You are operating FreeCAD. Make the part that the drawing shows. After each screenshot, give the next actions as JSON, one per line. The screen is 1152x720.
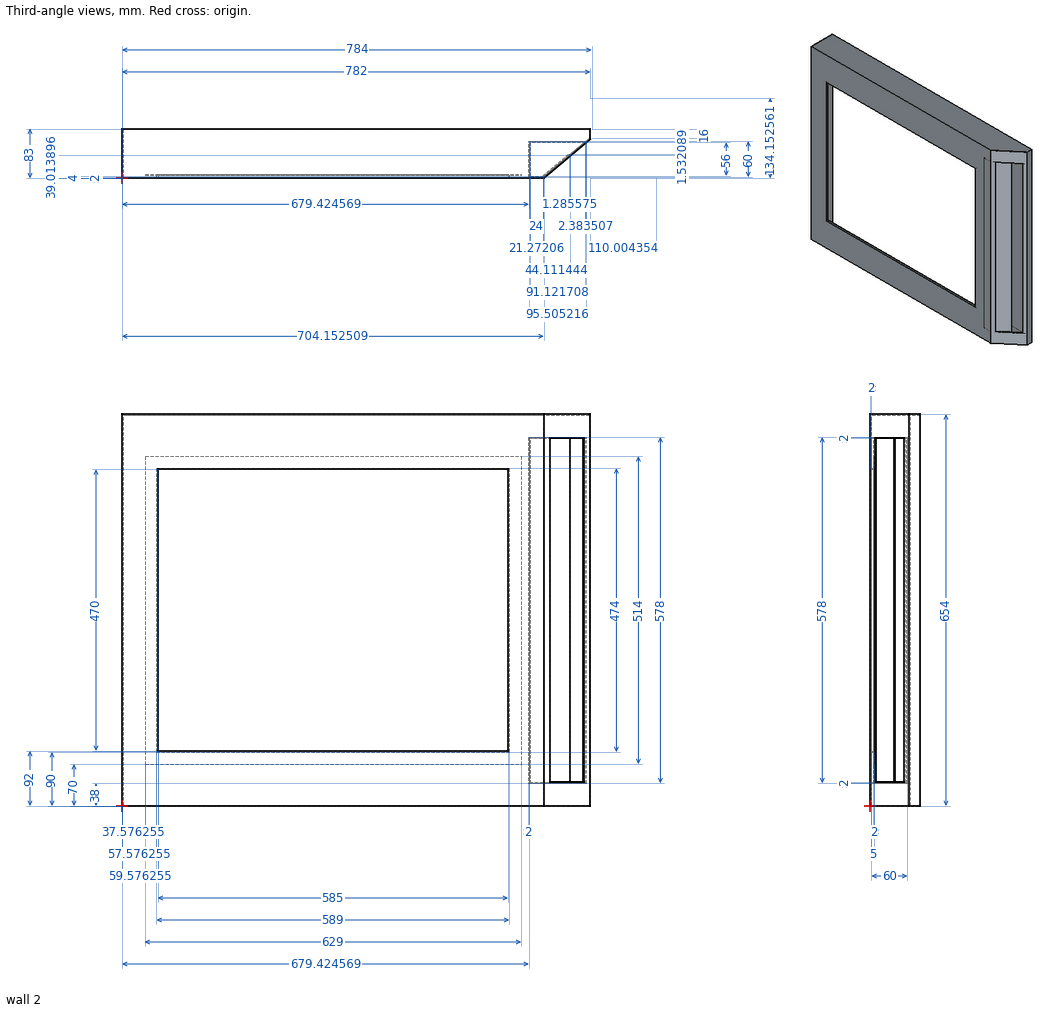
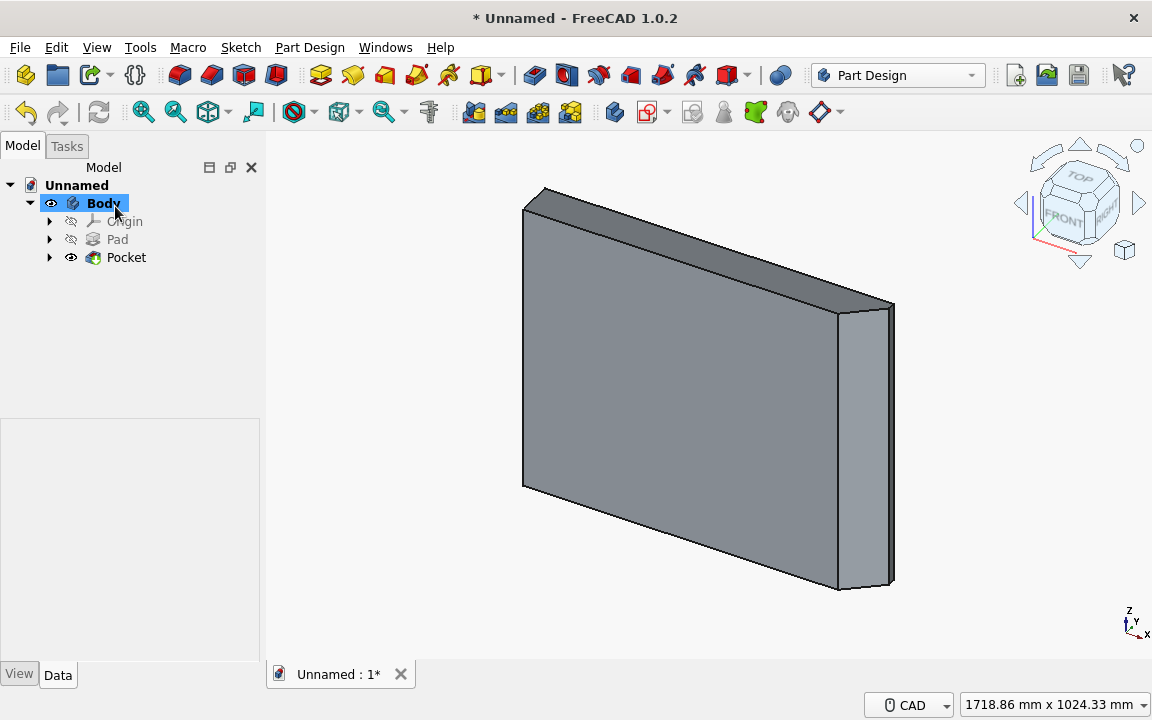
{"action": "key", "text": "0"}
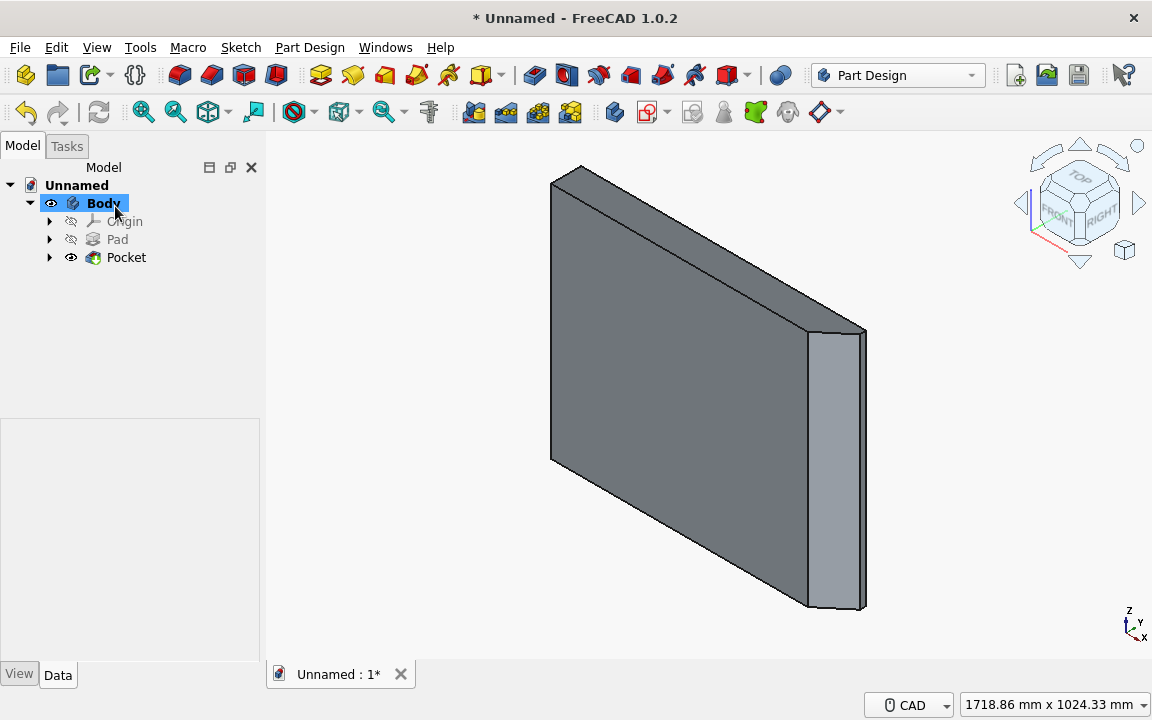
{"action": "key", "text": "2"}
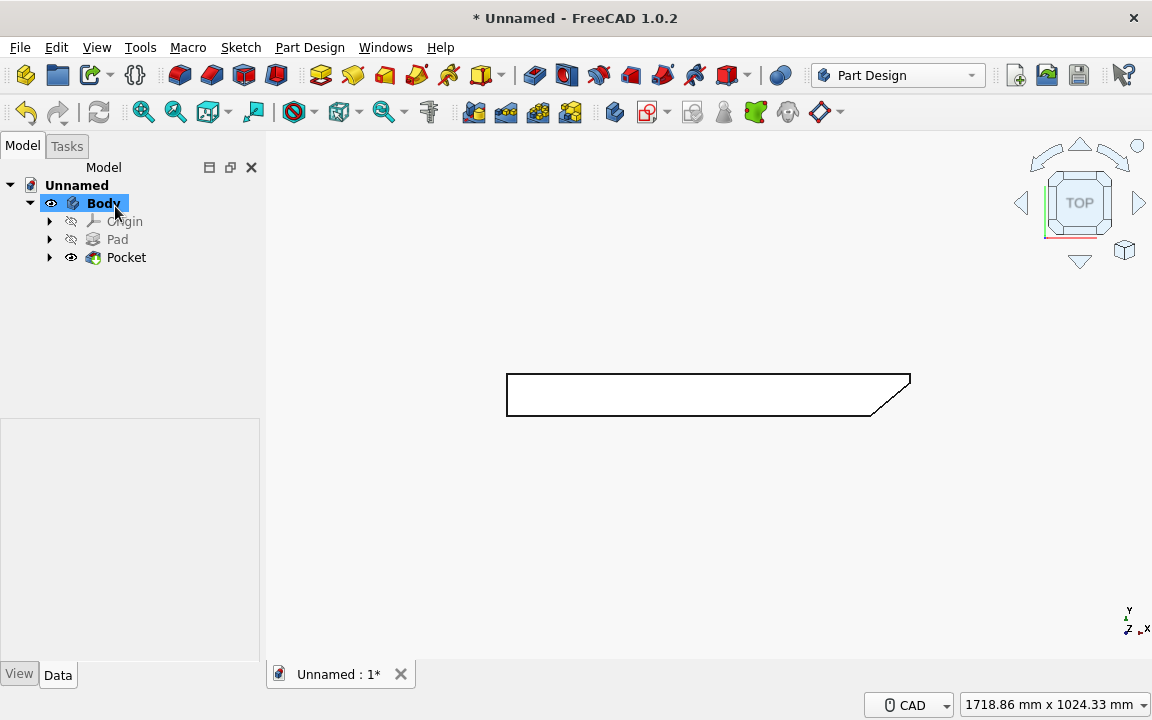
{"action": "key", "text": "1"}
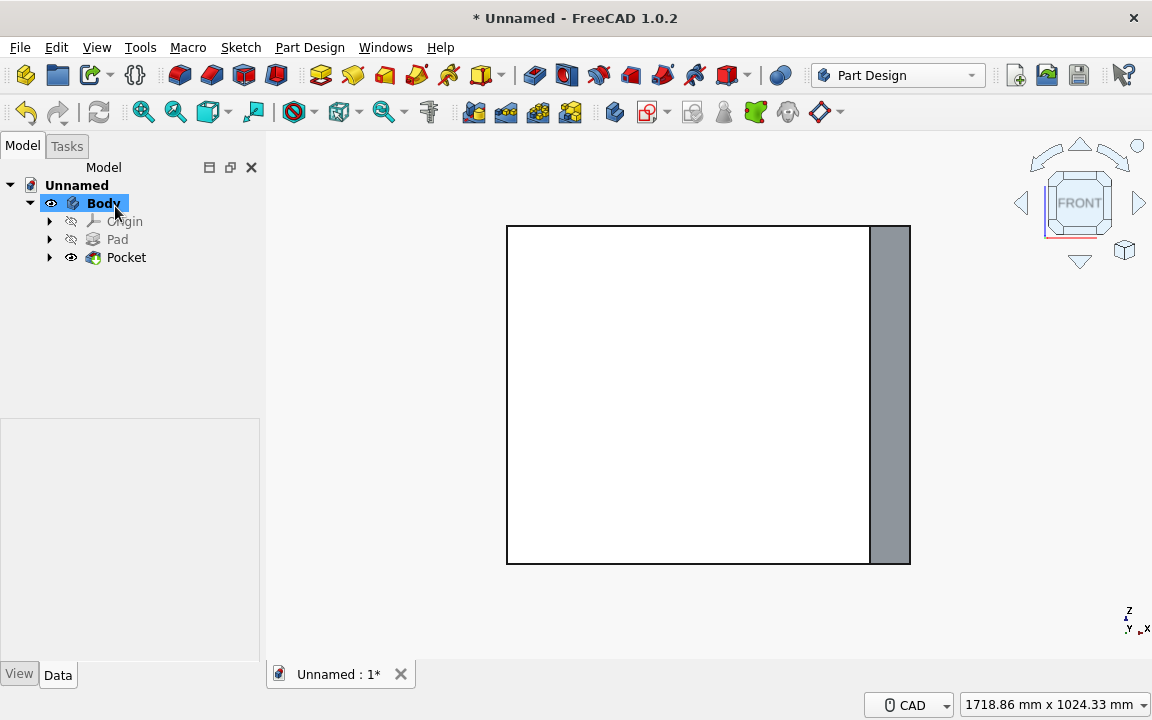
{"action": "key", "text": "3"}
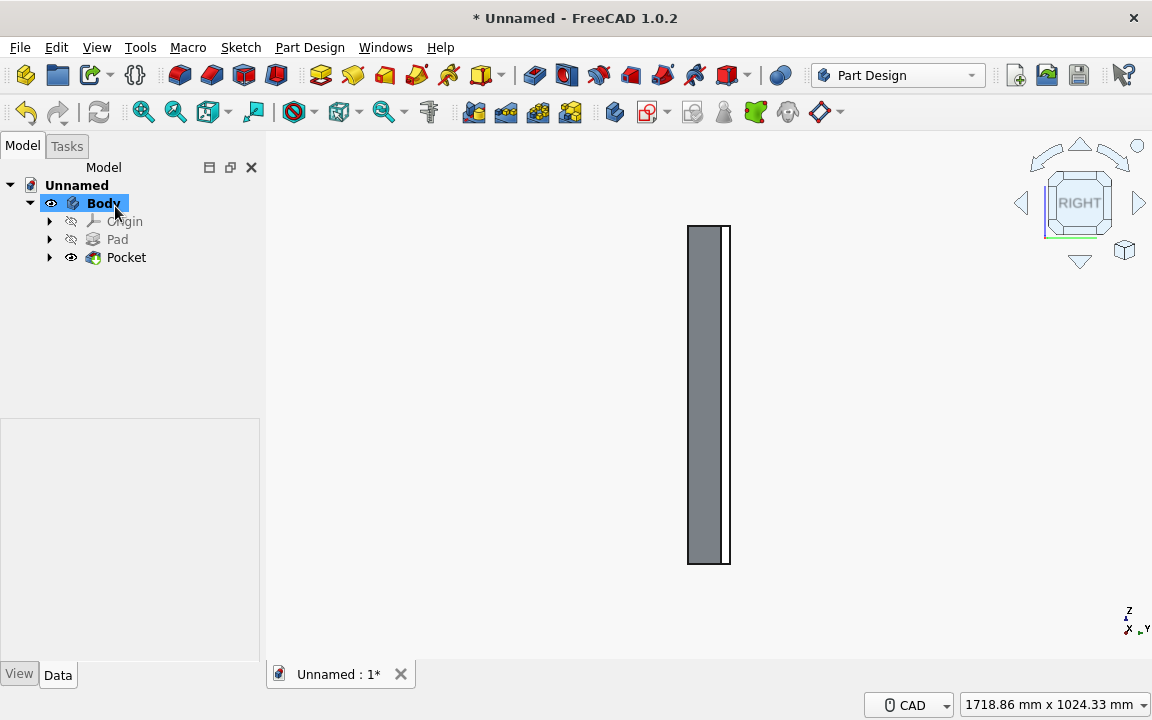
{"action": "key", "text": "5"}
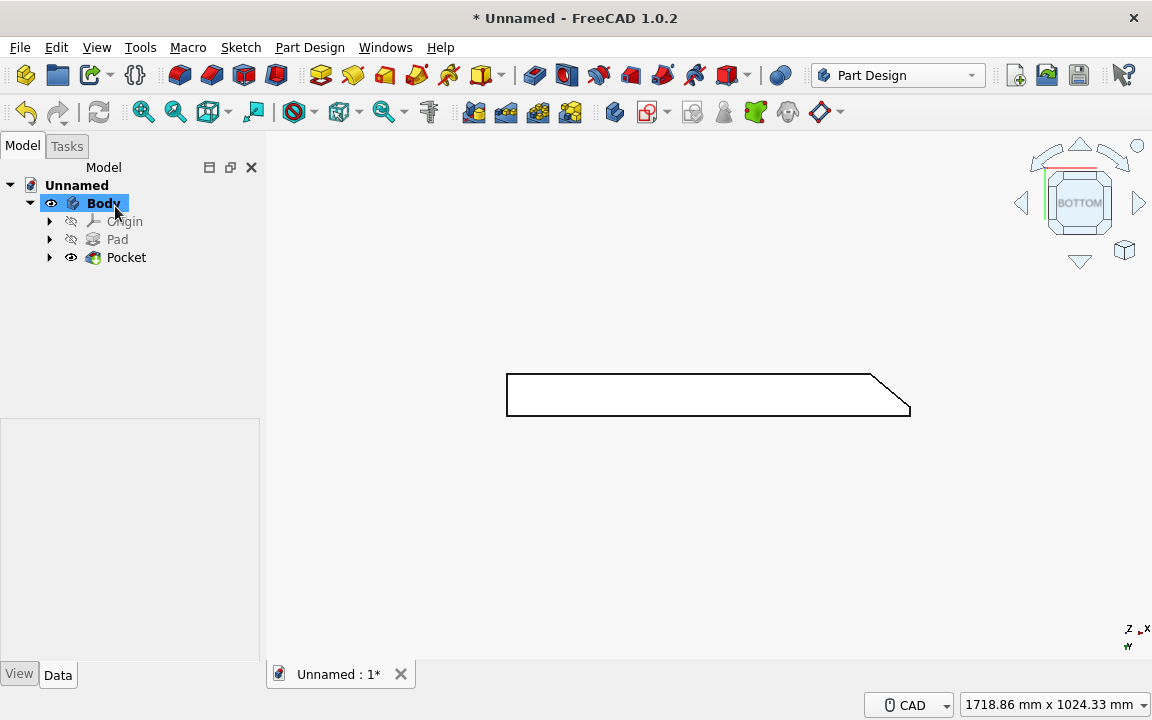
{"action": "key", "text": "4"}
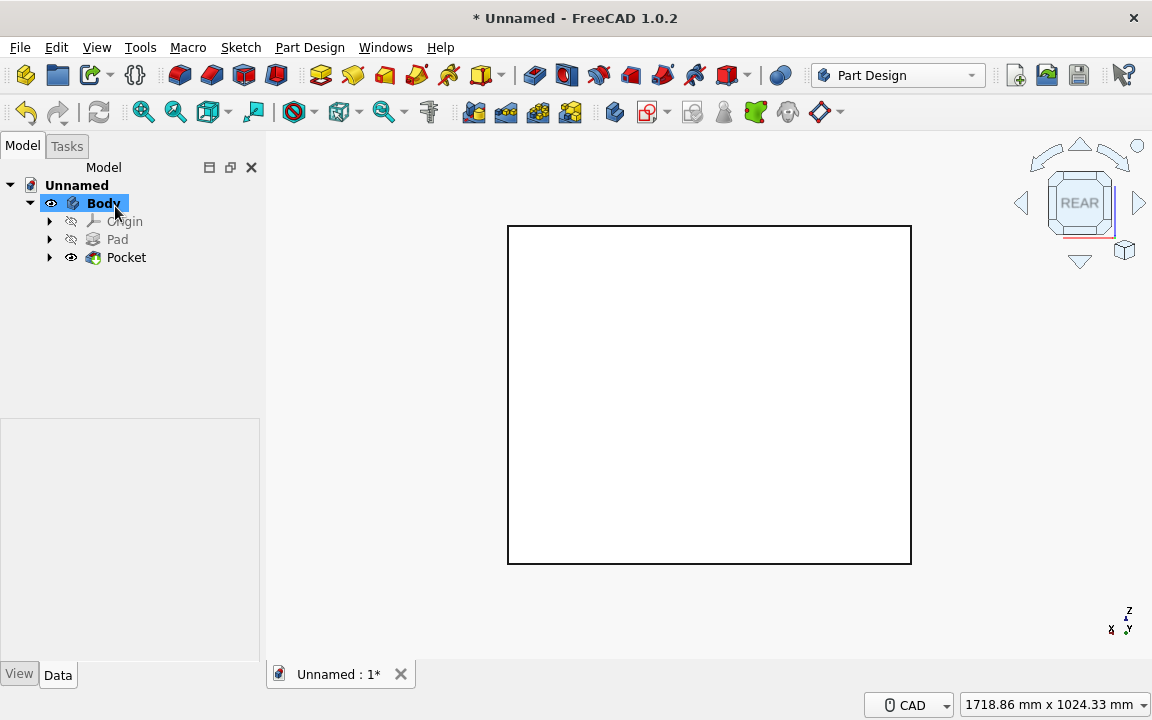
{"action": "left_click", "coordinate": [710, 394]}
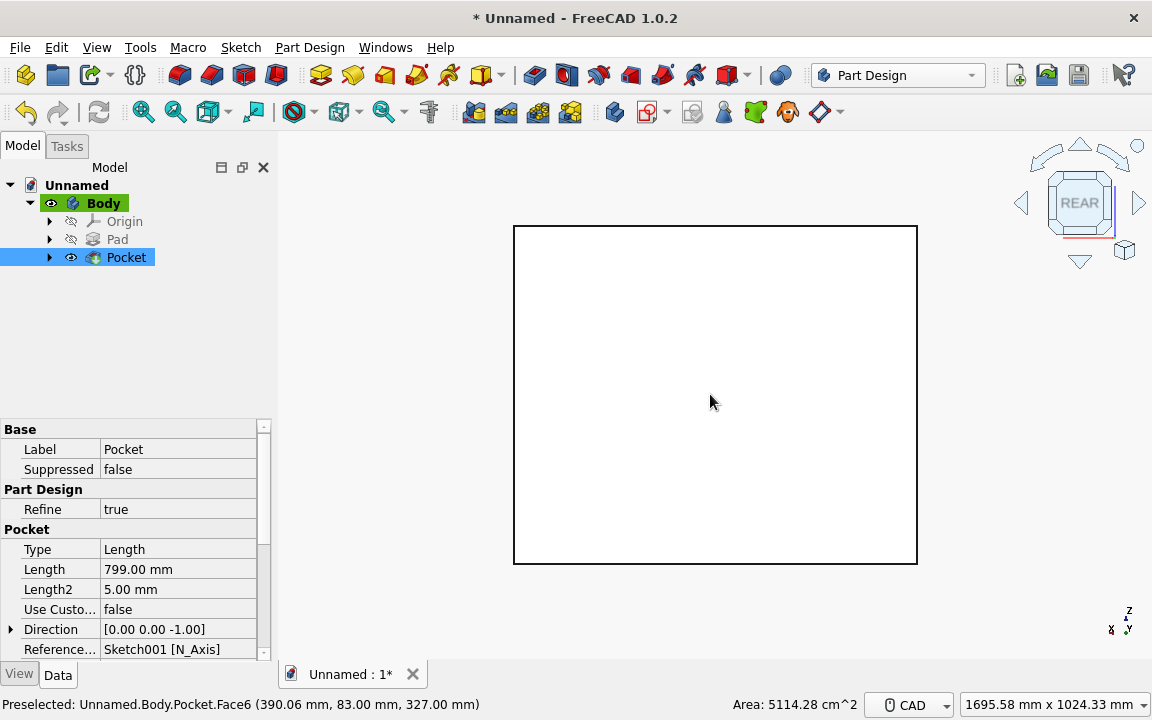
{"action": "left_click", "coordinate": [276, 76]}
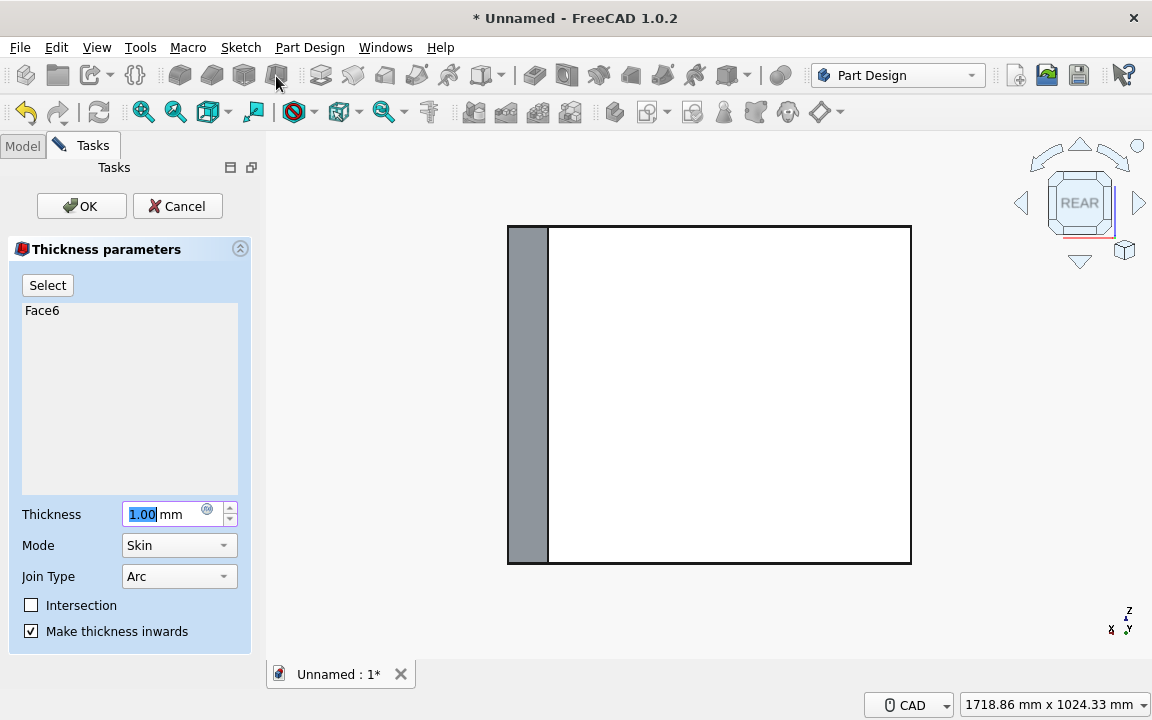
{"action": "type", "text": "2"}
{"action": "key", "text": "Tab"}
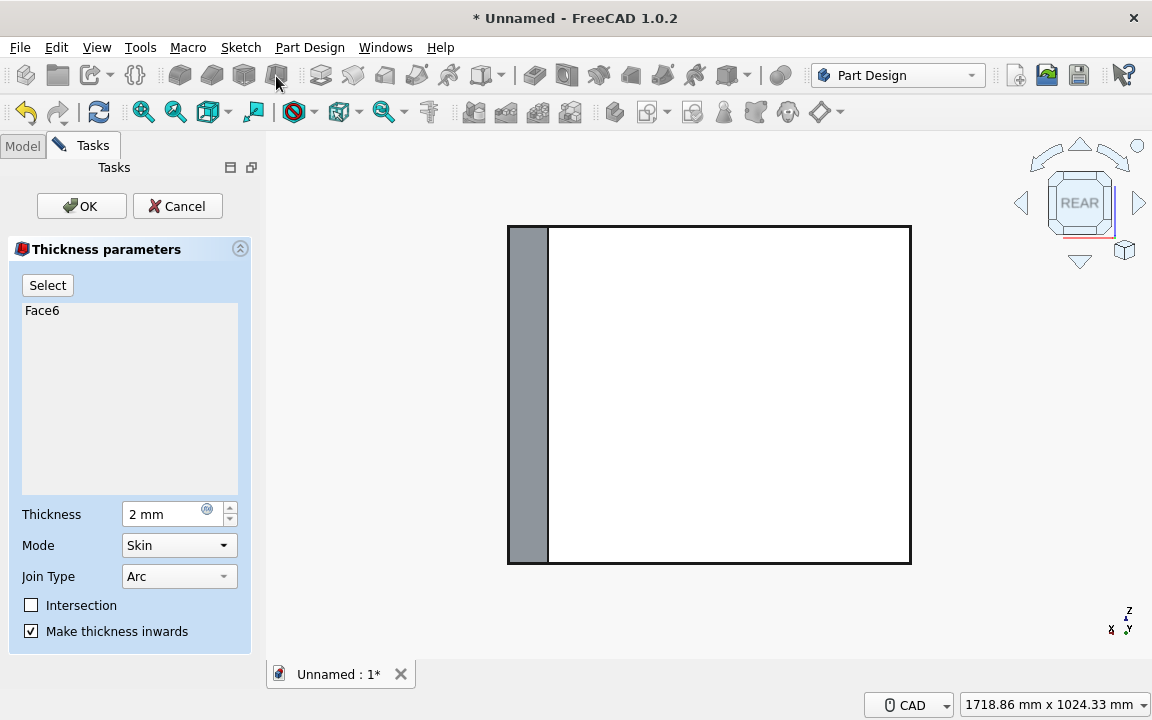
{"action": "left_click", "coordinate": [180, 576]}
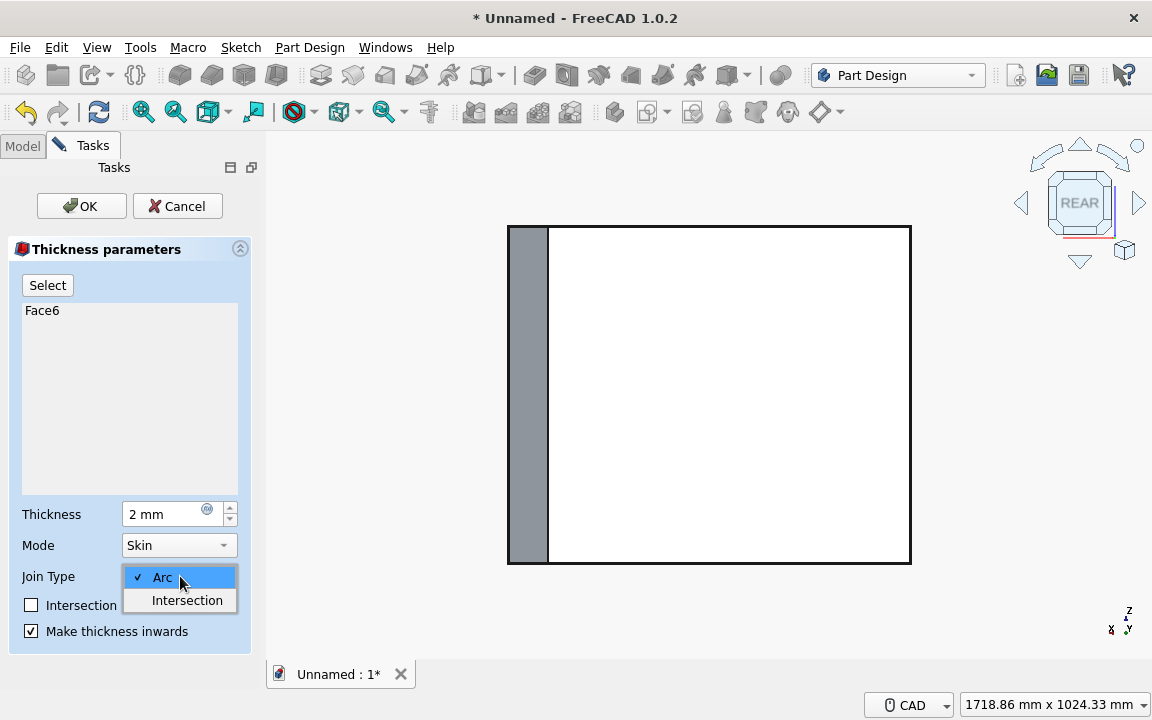
{"action": "left_click", "coordinate": [179, 600]}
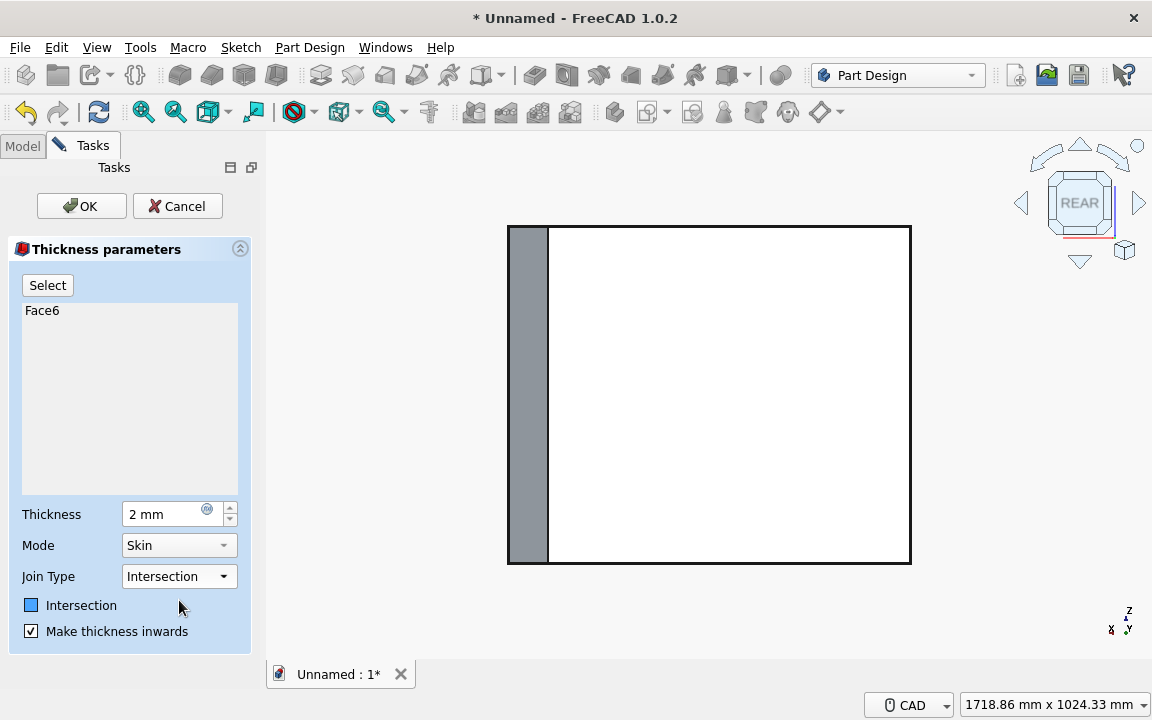
{"action": "left_click", "coordinate": [82, 206]}